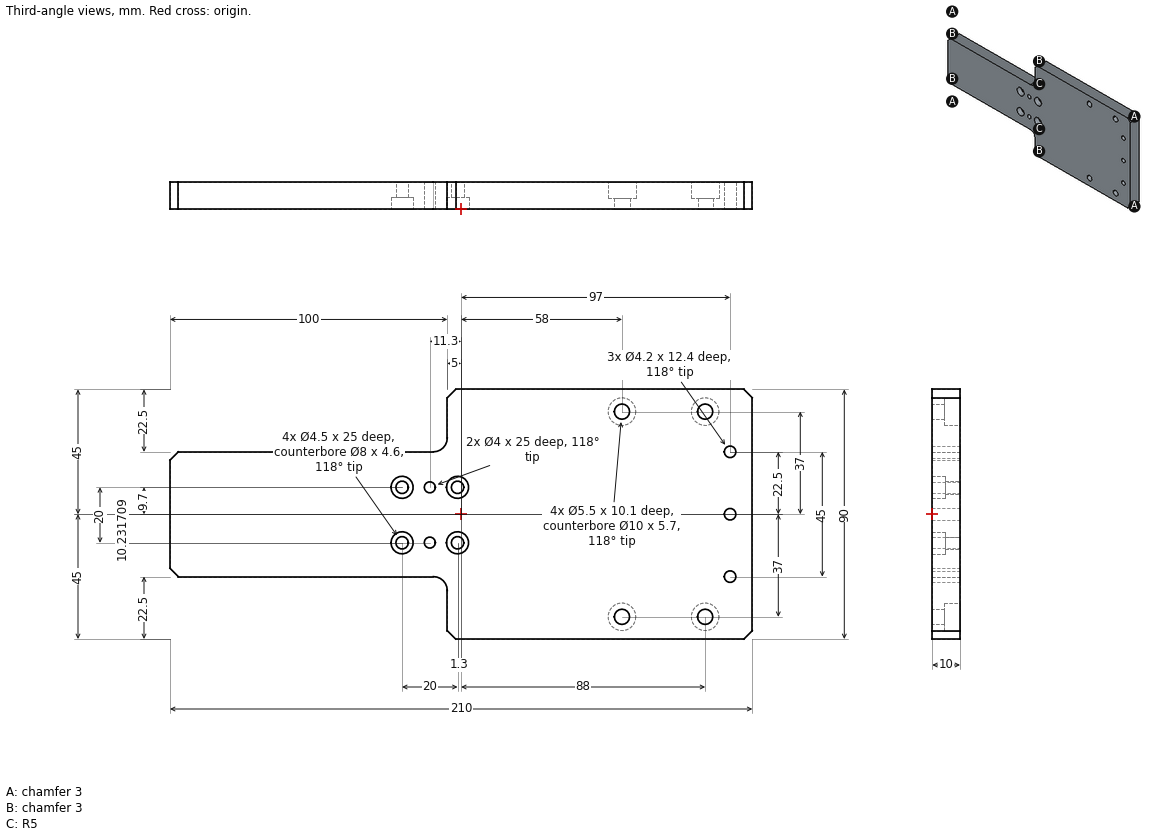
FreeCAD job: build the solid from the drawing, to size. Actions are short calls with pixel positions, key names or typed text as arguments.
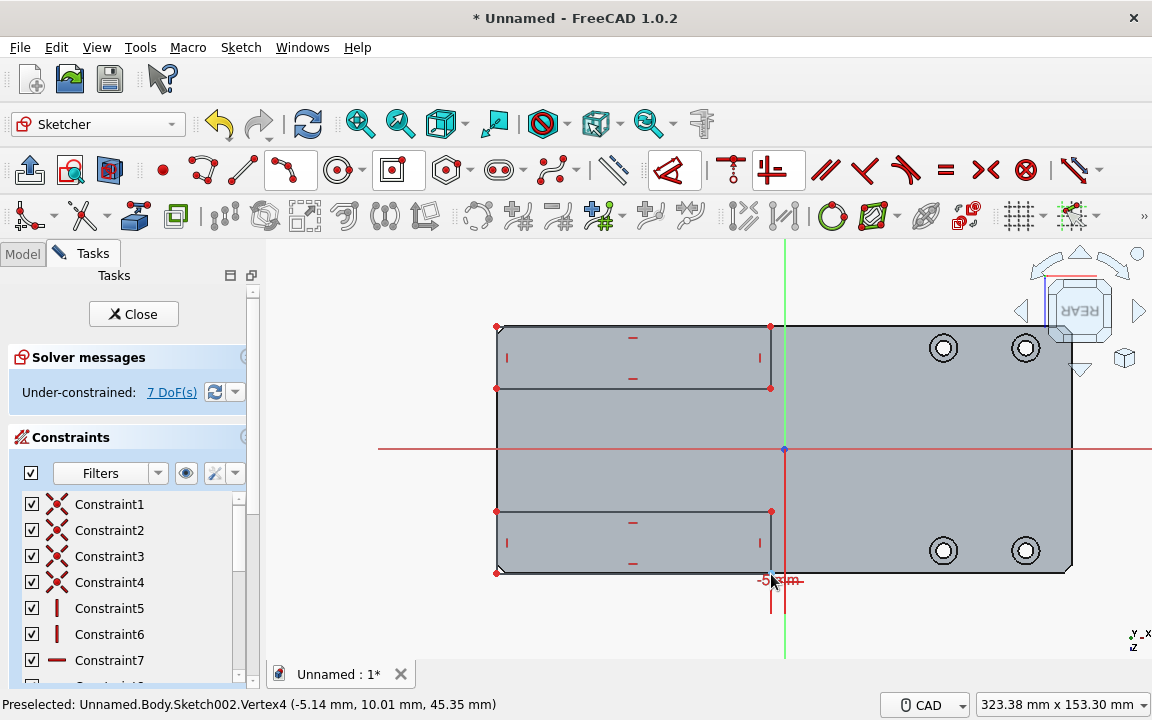
scroll(771, 389, up, 6)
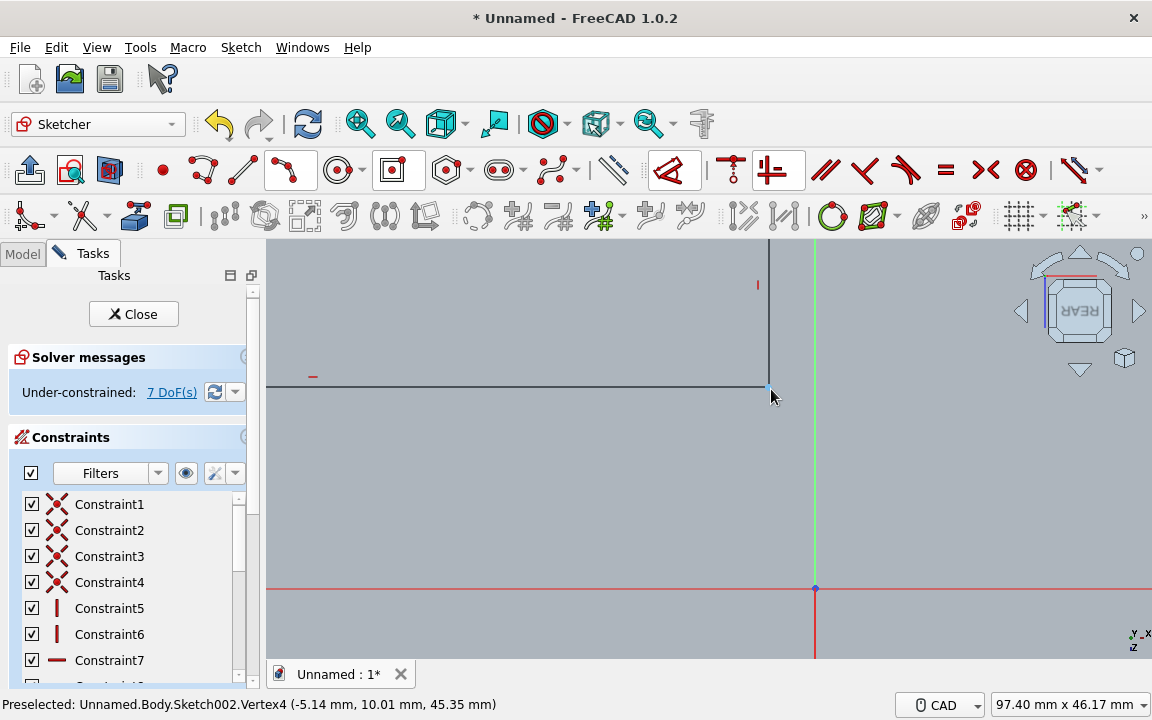
click(769, 387)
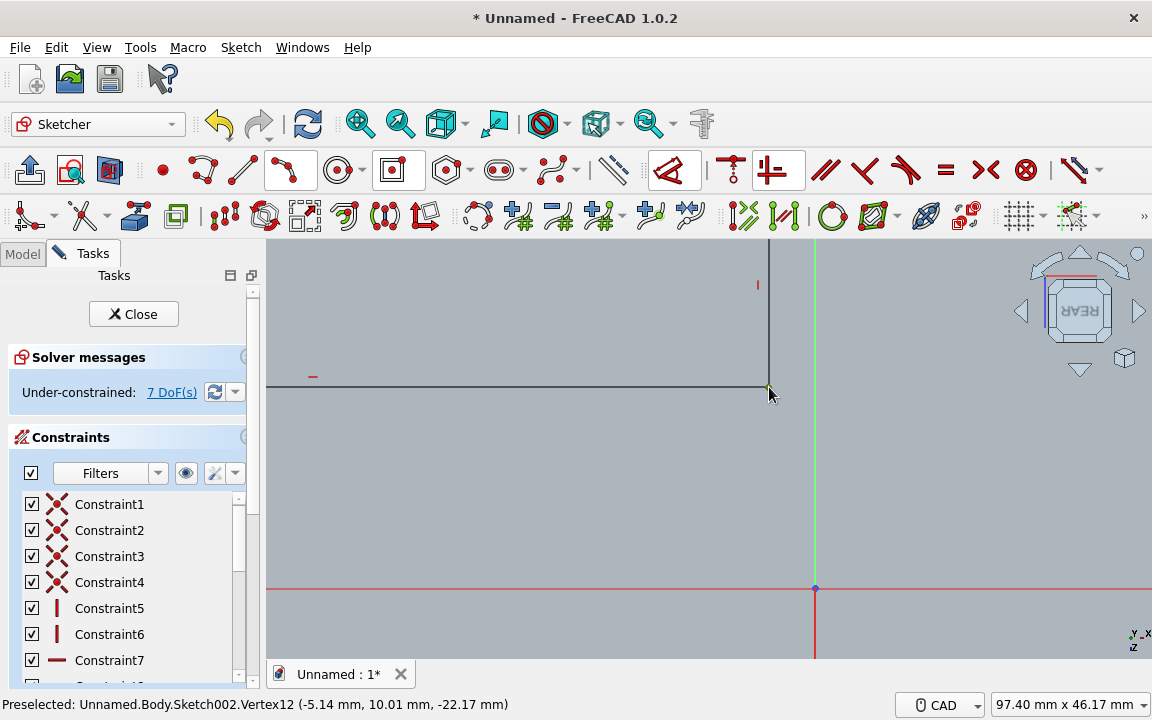
click(696, 170)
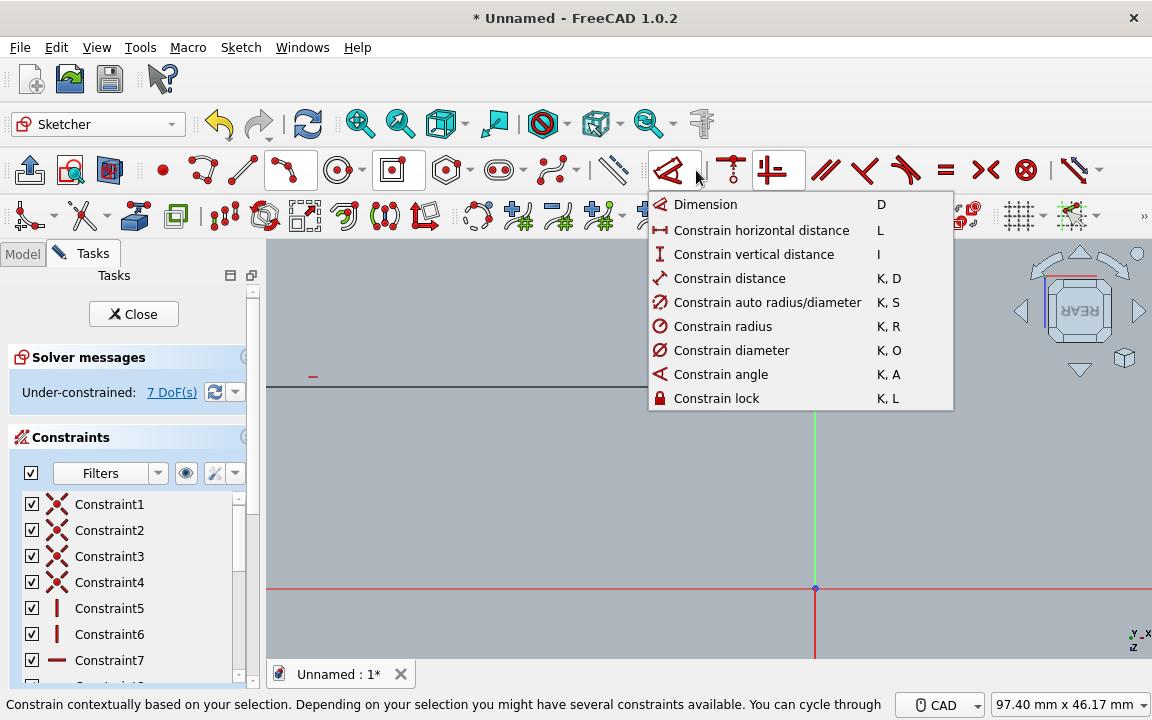
click(801, 230)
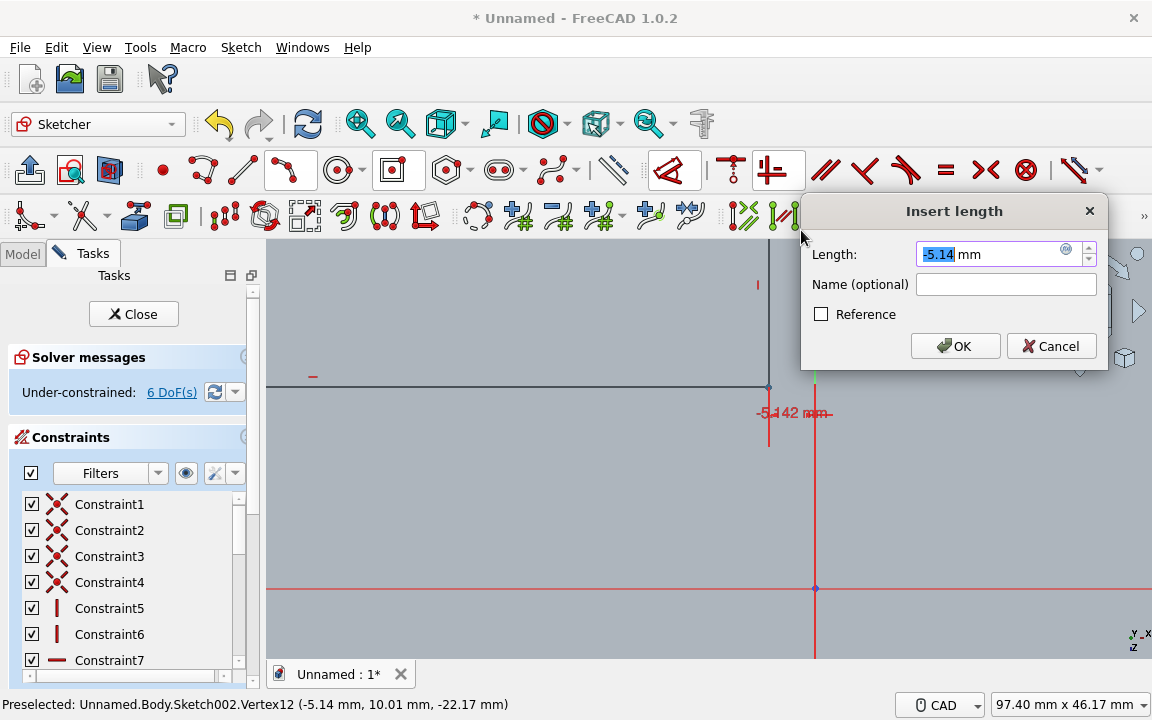
text(-5)
key(Return)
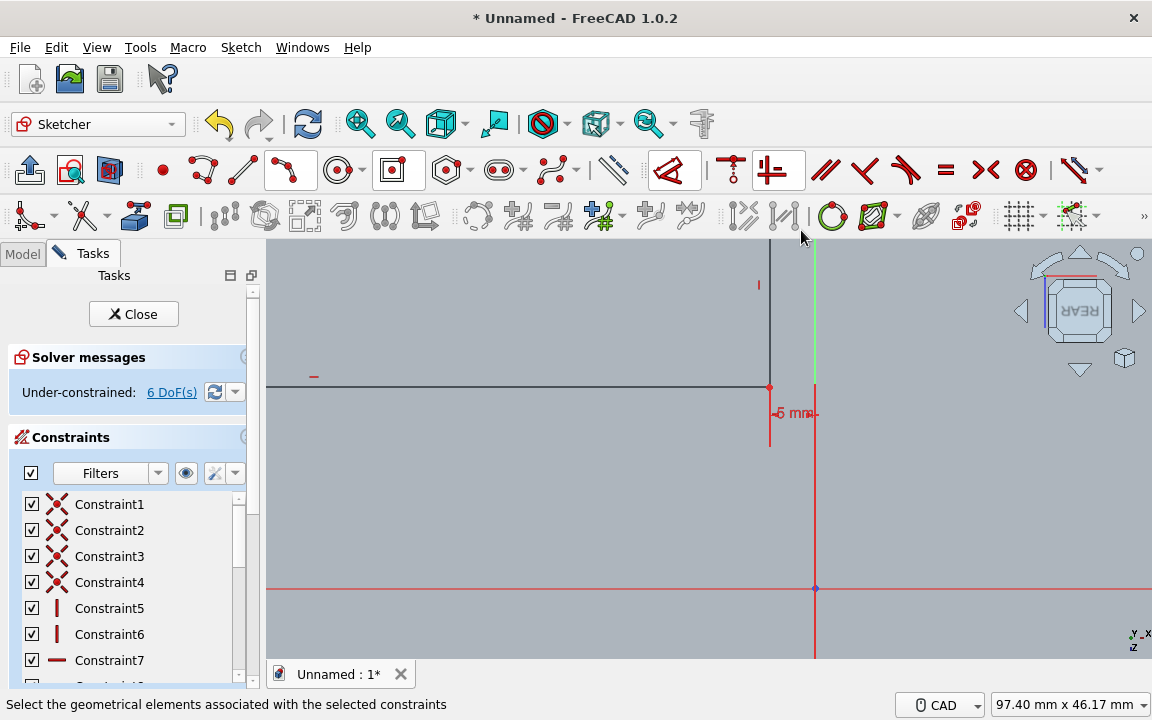
scroll(771, 389, down, 6)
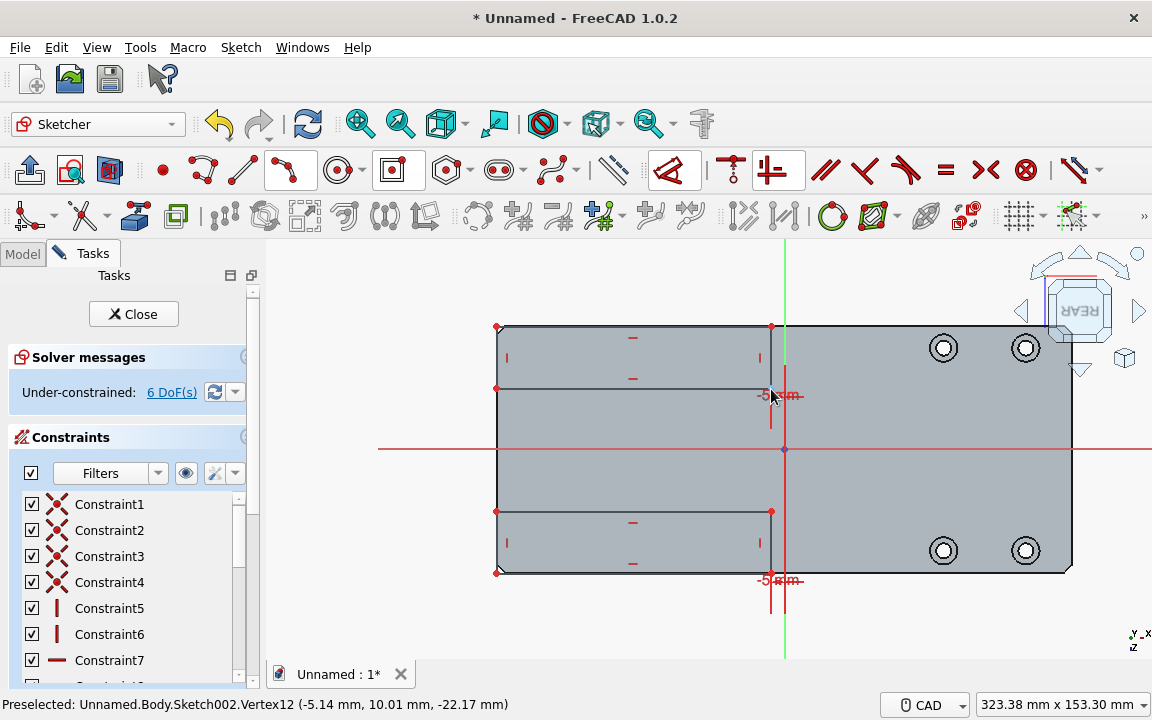
click(579, 574)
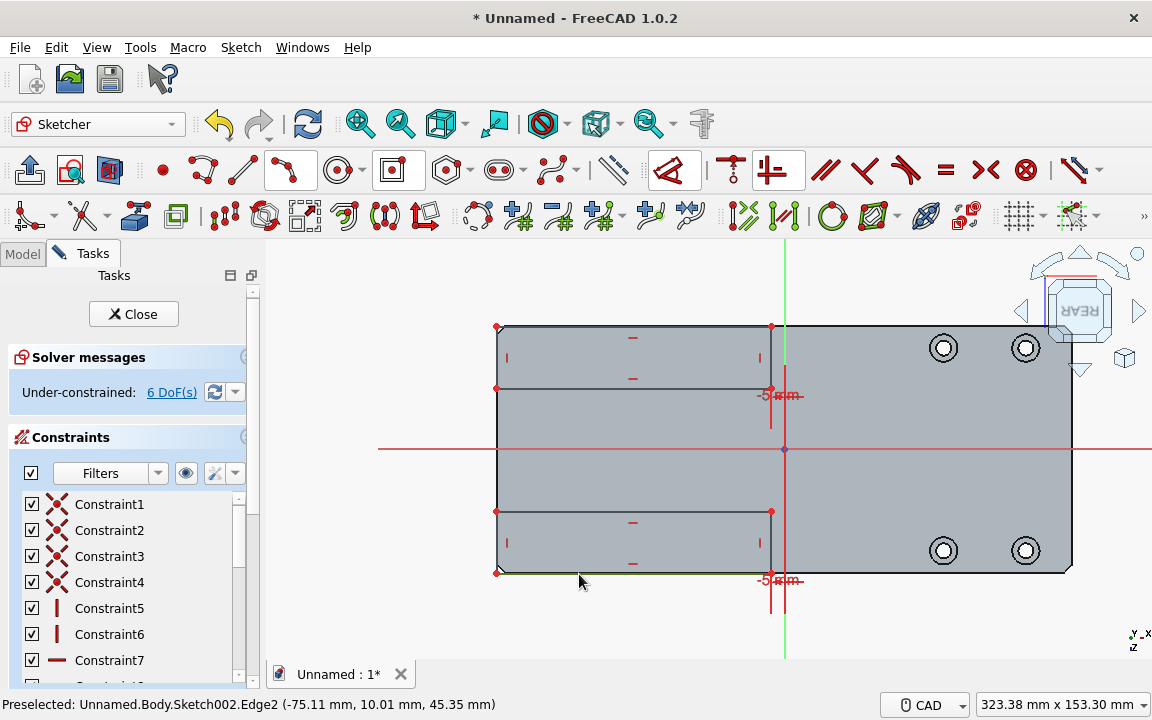
key(l)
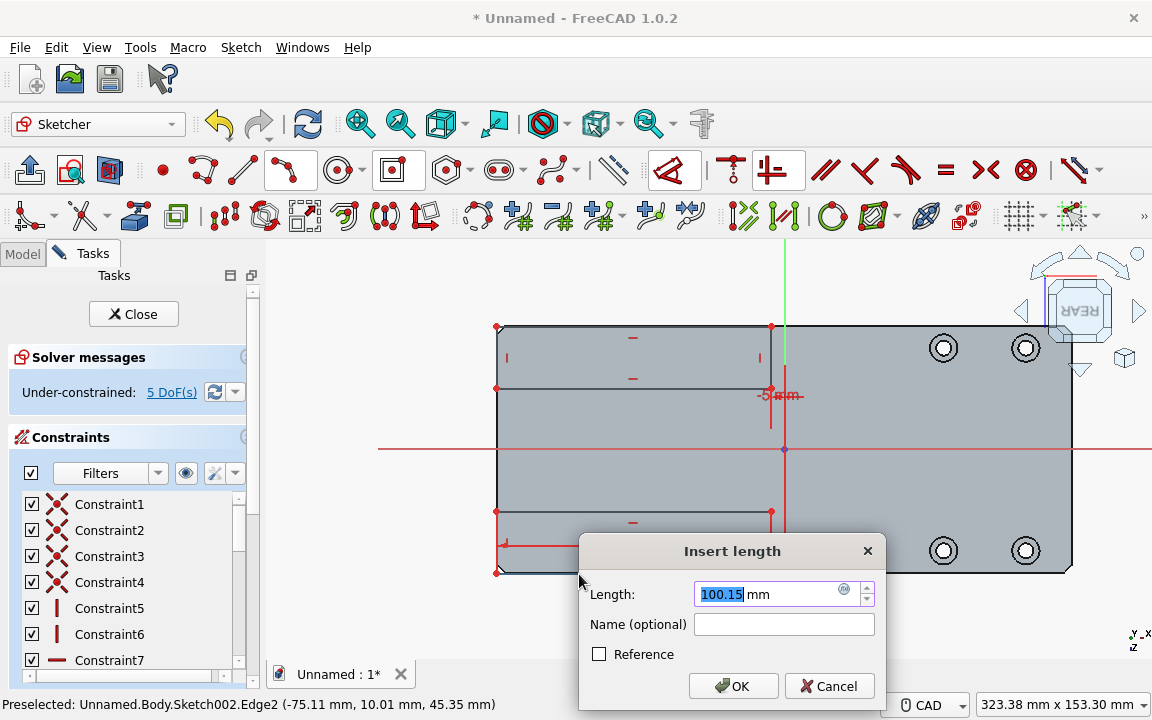
text(100)
key(Return)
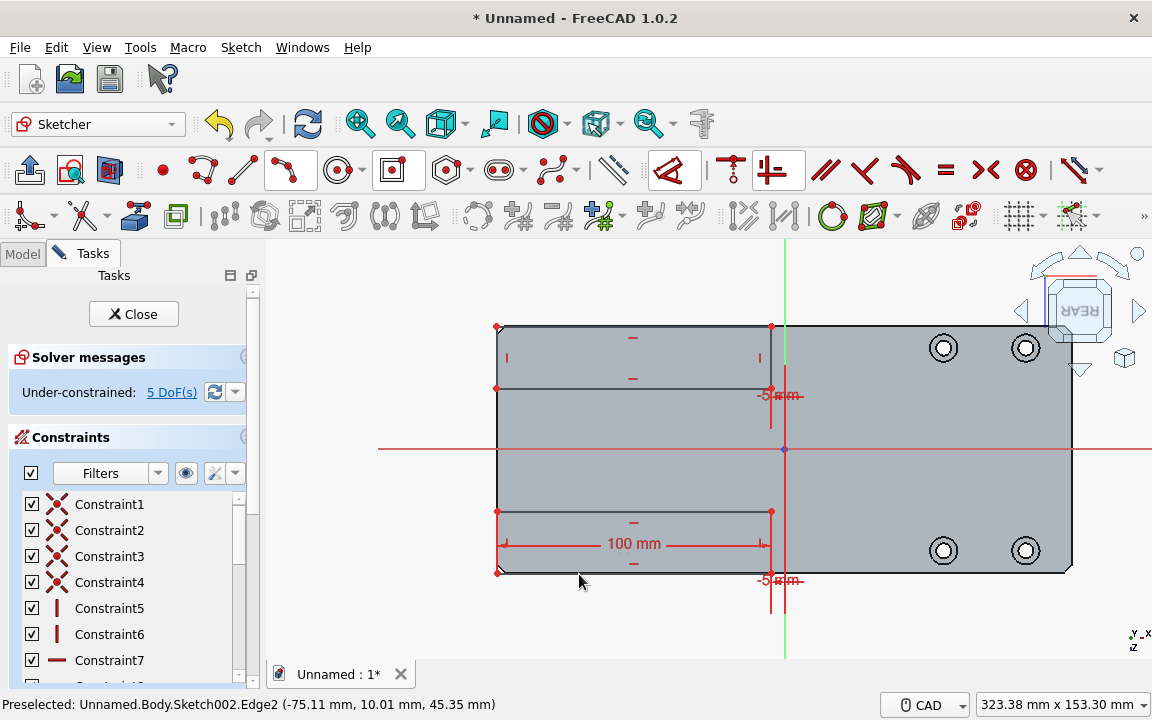
click(579, 389)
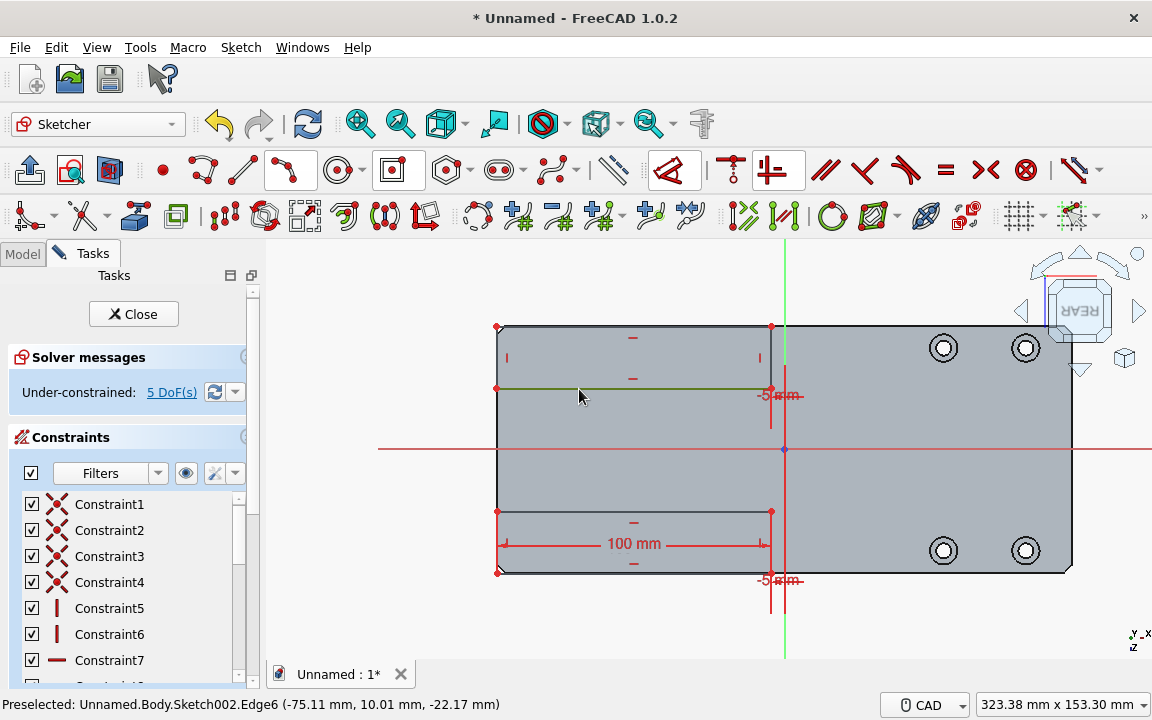
key(l)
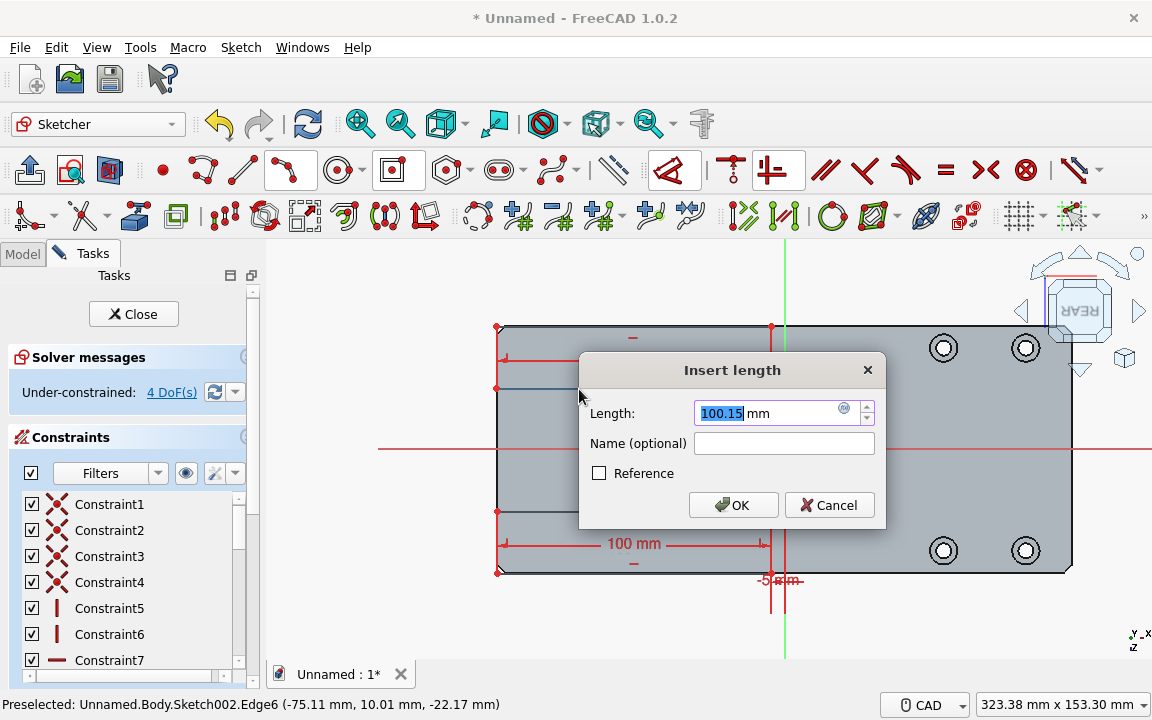
text(100)
key(Return)